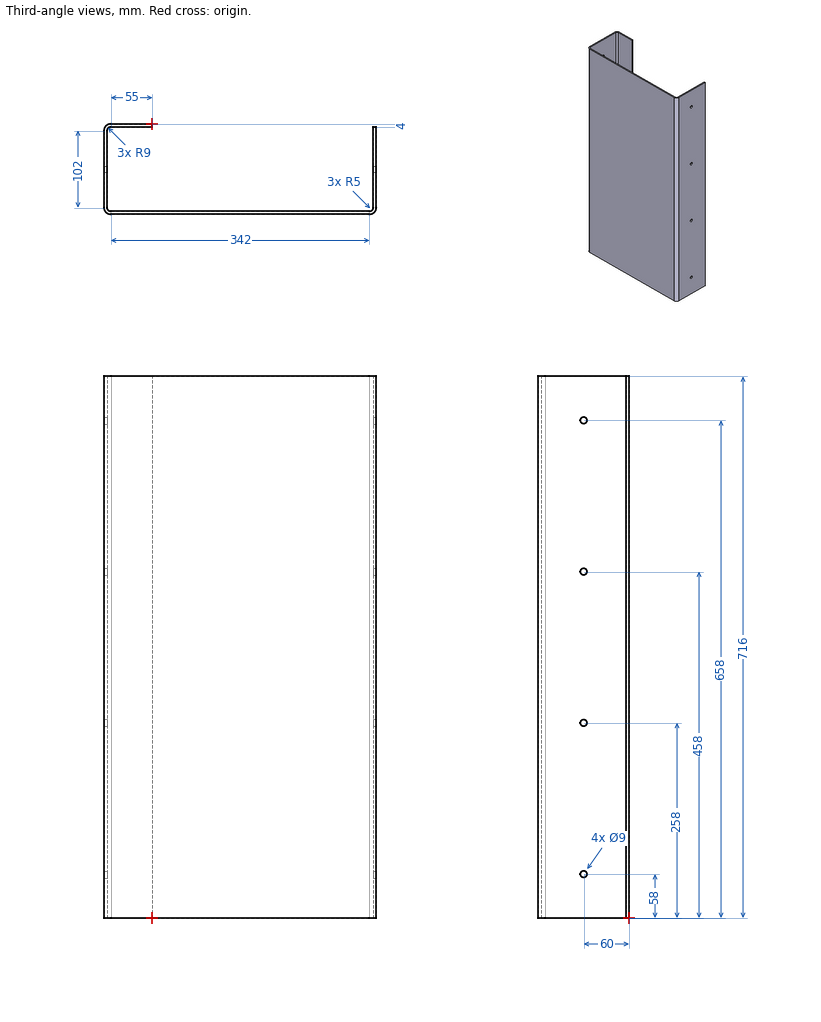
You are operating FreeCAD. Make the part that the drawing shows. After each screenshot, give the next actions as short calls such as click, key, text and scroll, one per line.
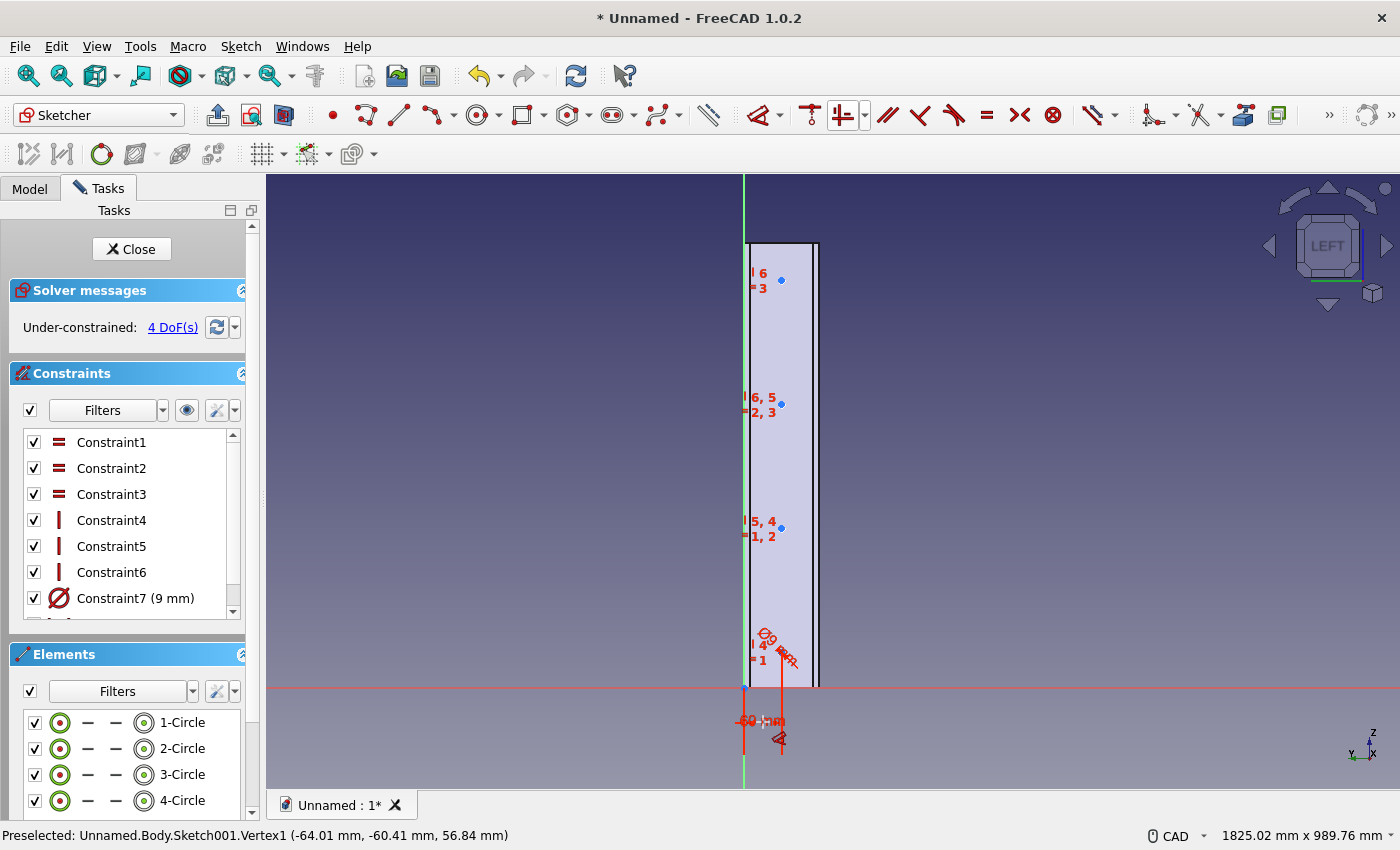
click(782, 653)
click(710, 671)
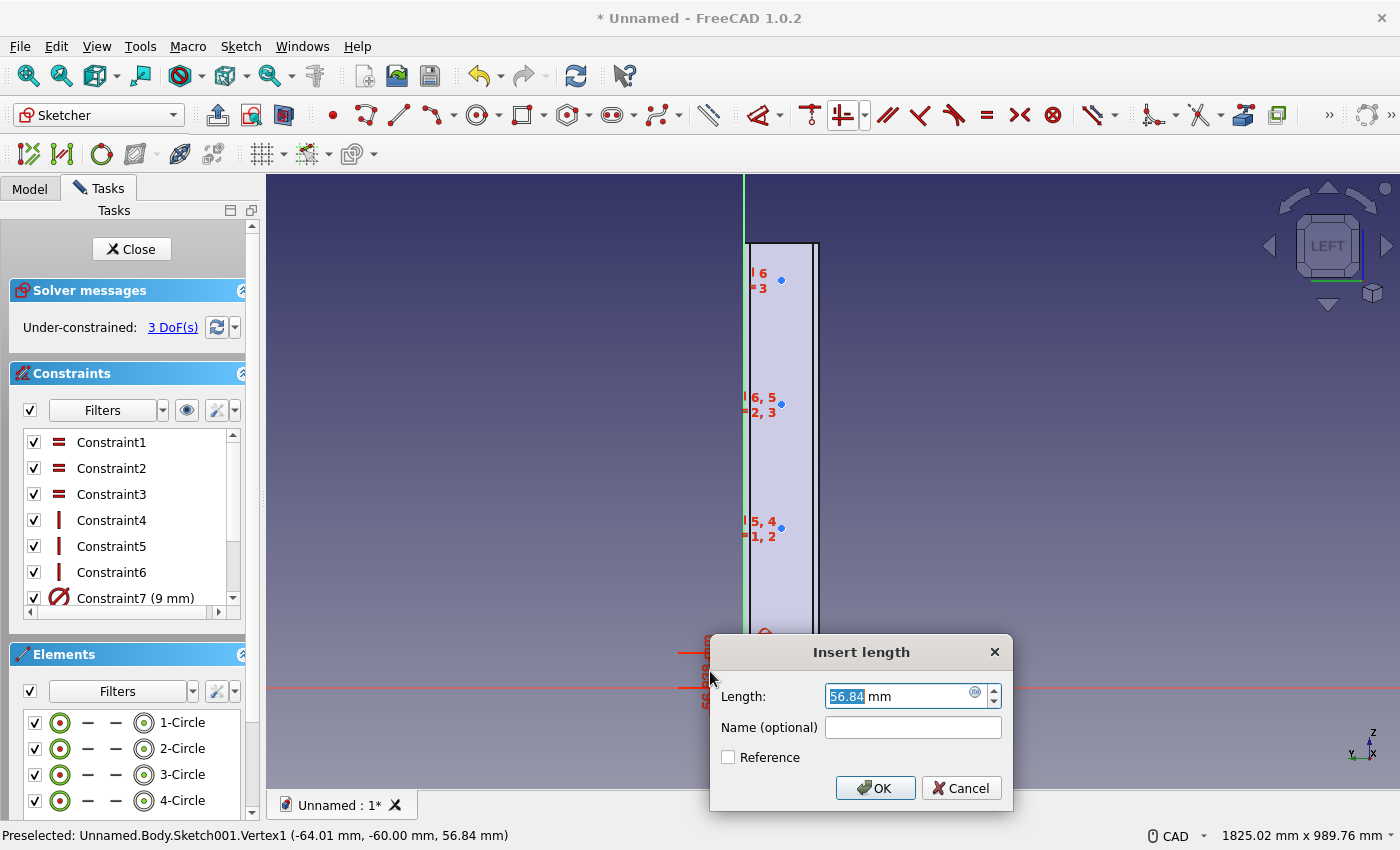
text(58)
key(Return)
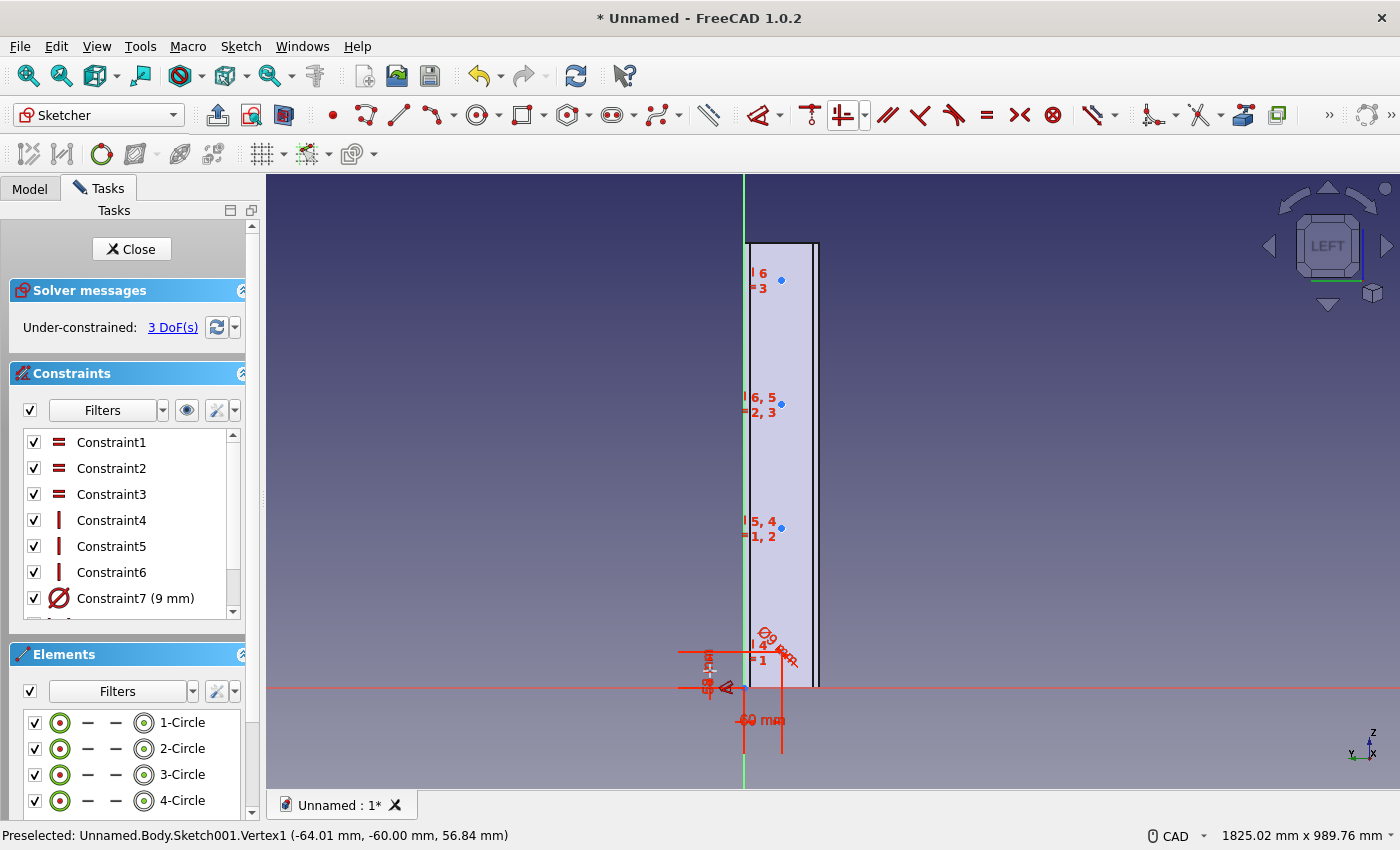
click(782, 529)
click(710, 609)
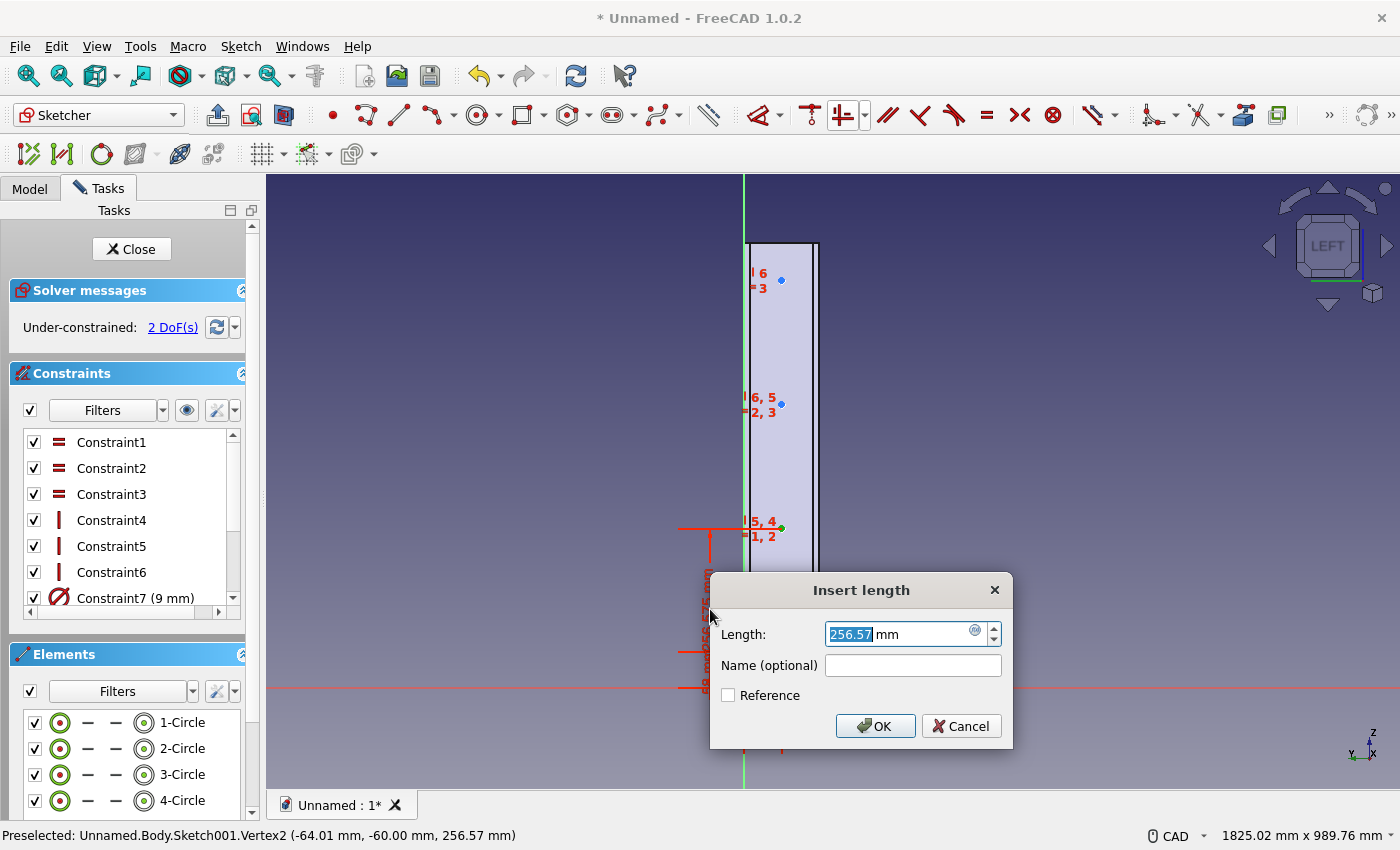
text(258)
key(Return)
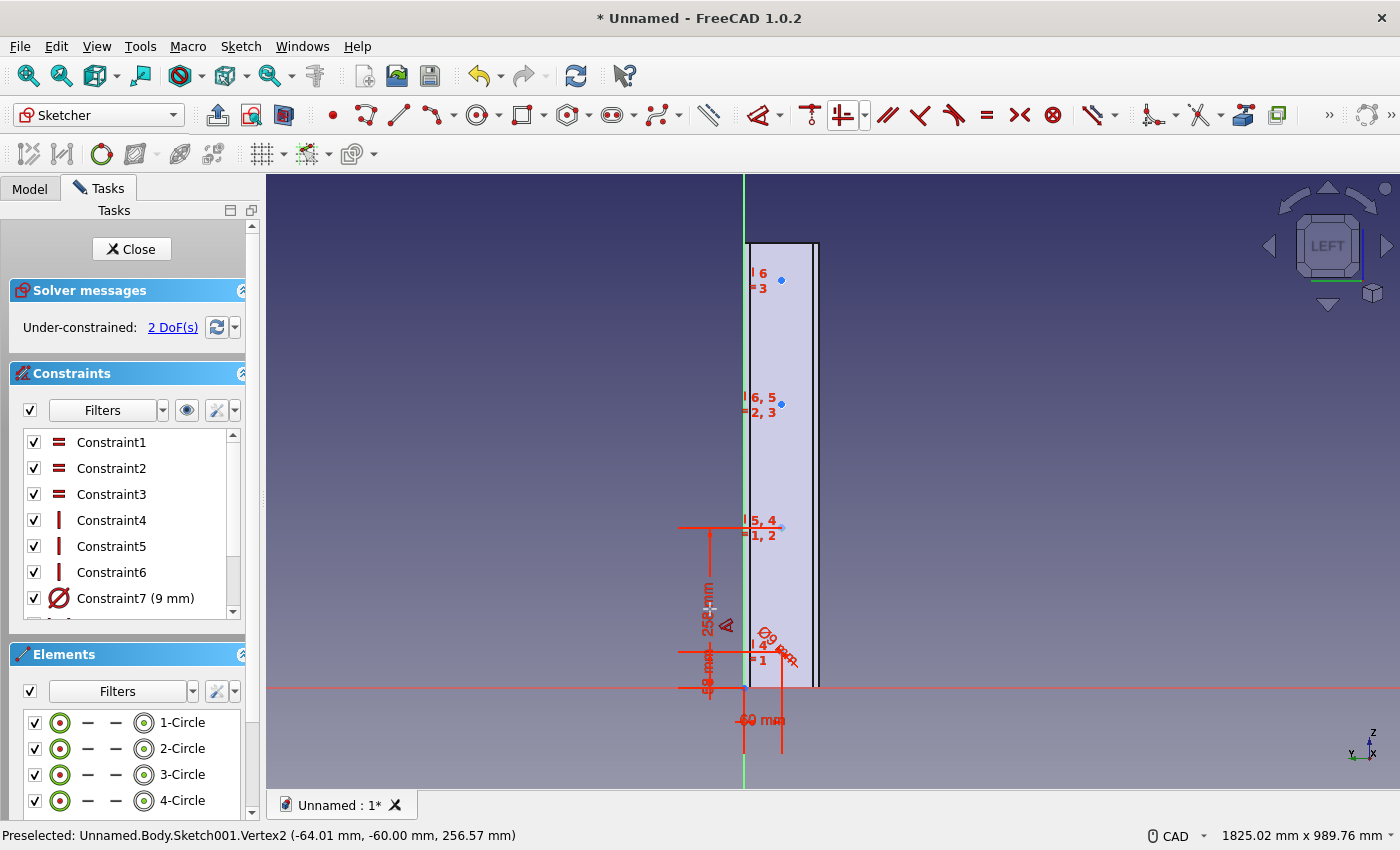
click(782, 405)
click(710, 547)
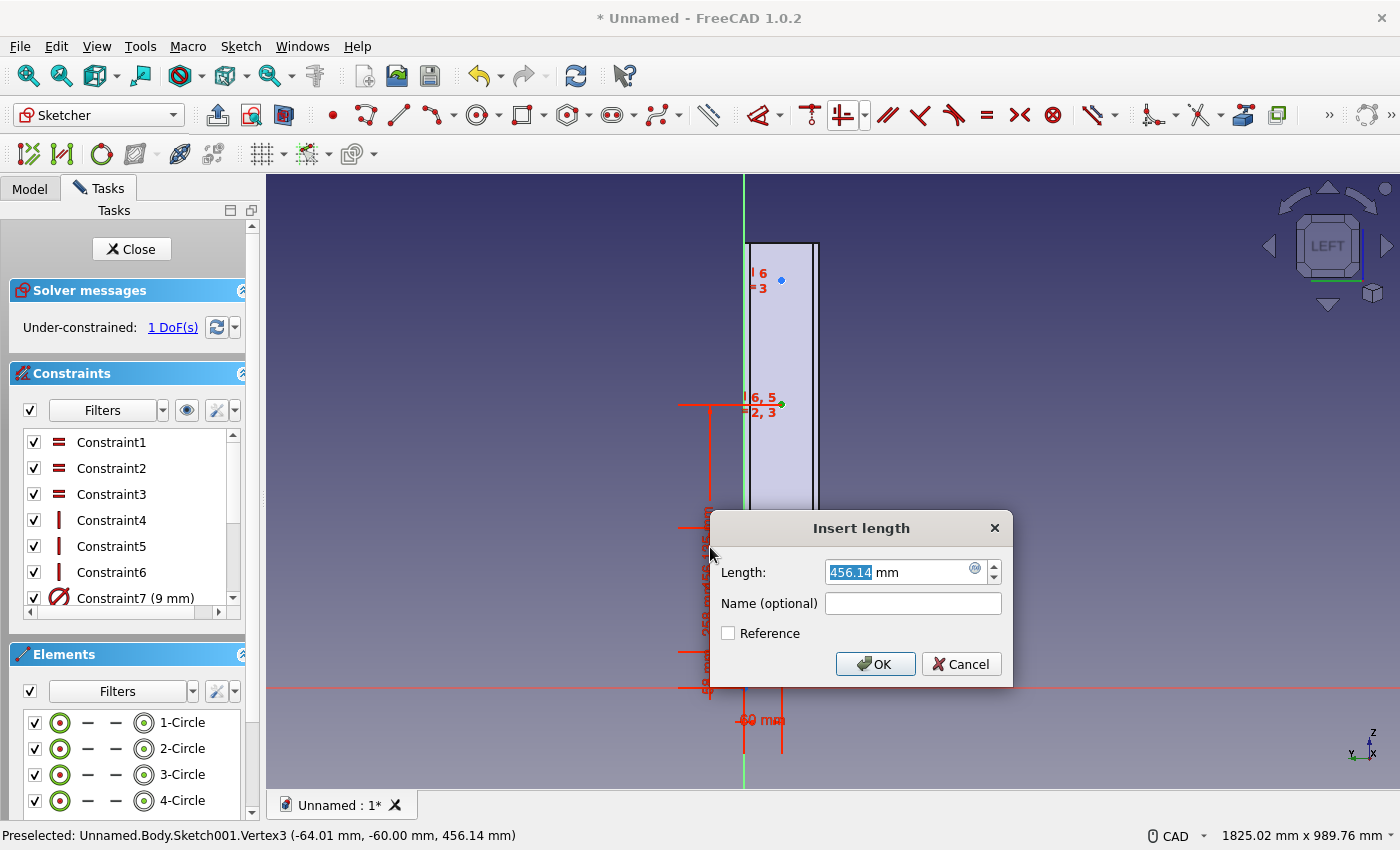
text(458)
key(Return)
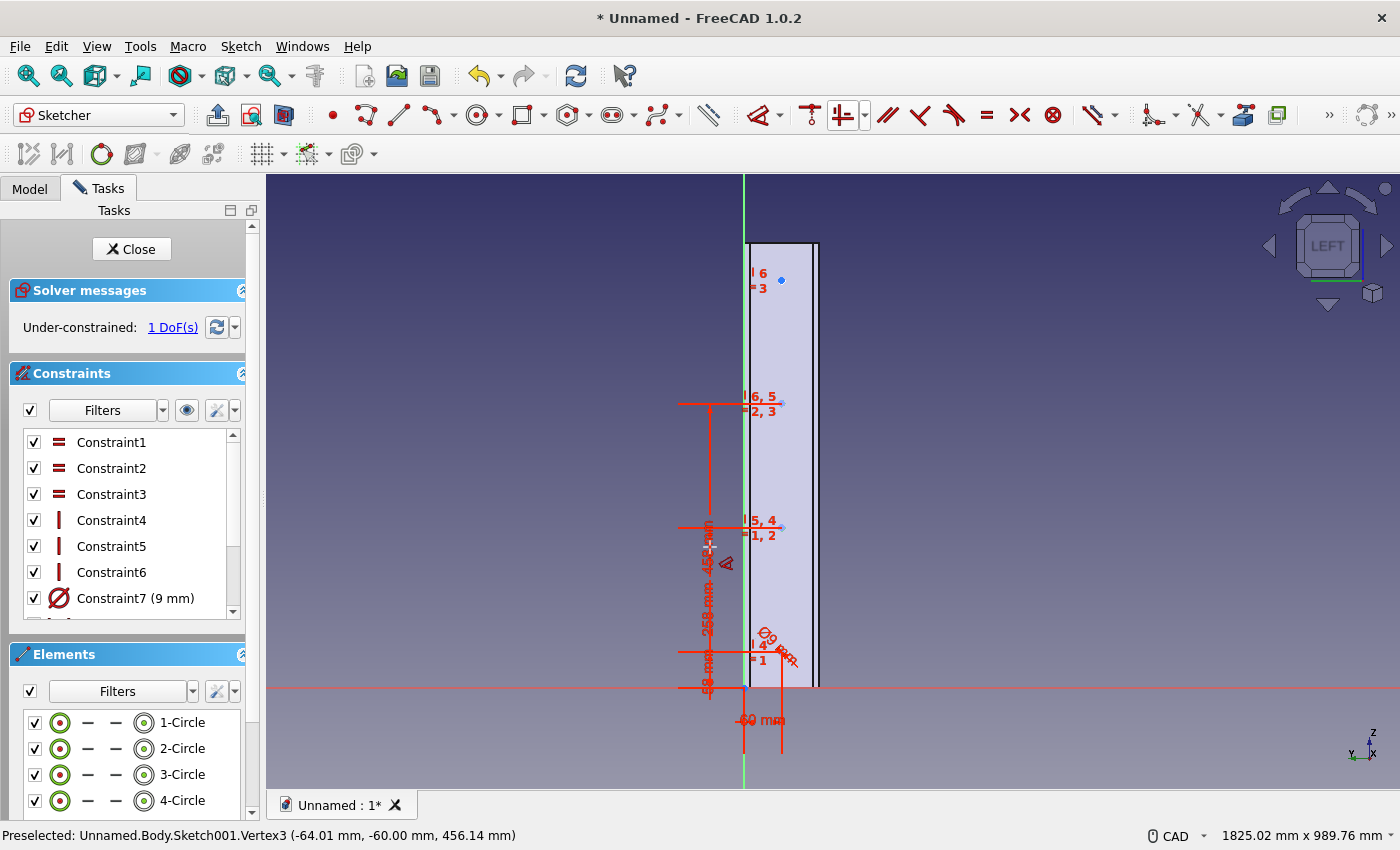
click(782, 281)
click(710, 485)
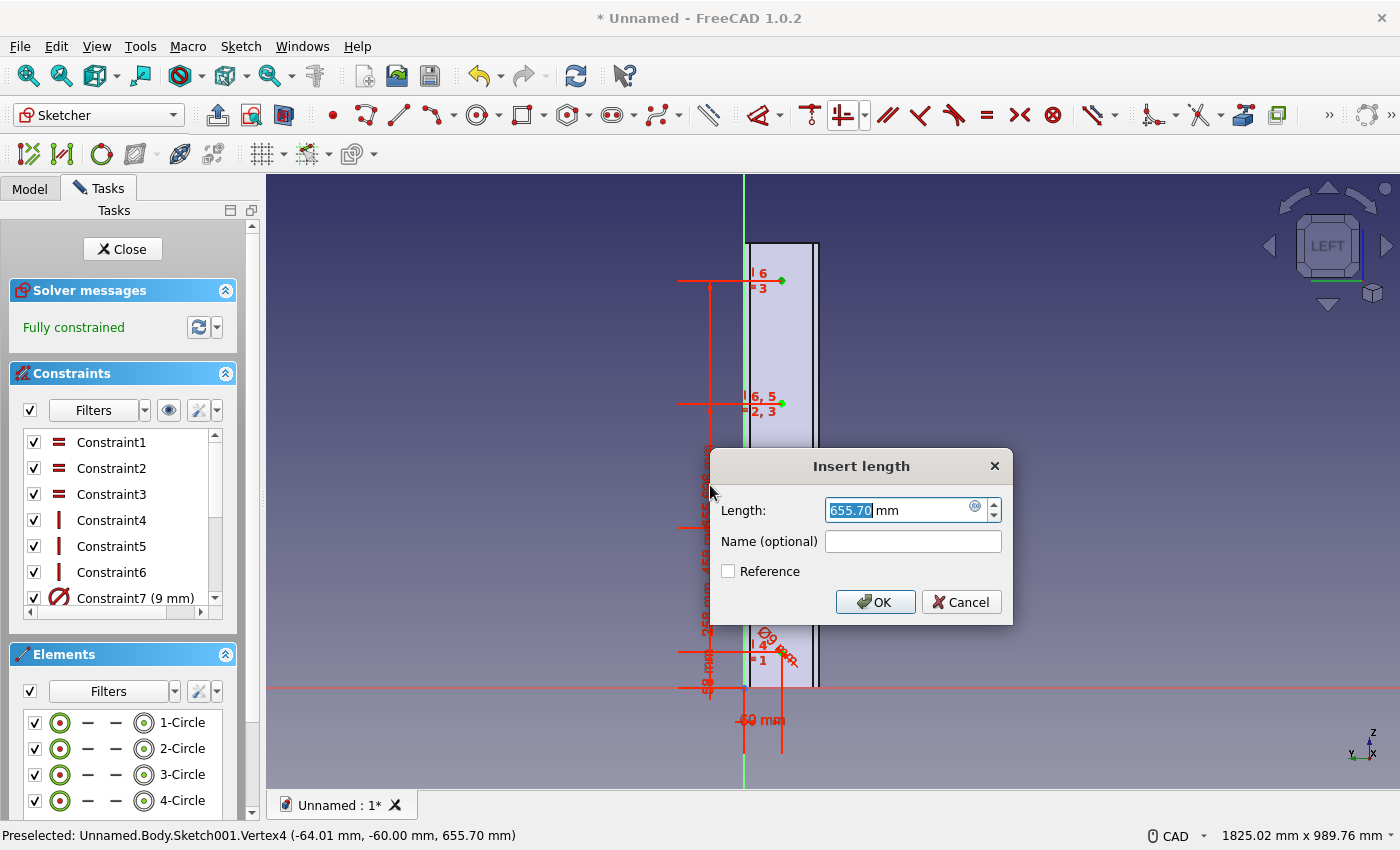
text(658)
key(Return)
key(Escape)